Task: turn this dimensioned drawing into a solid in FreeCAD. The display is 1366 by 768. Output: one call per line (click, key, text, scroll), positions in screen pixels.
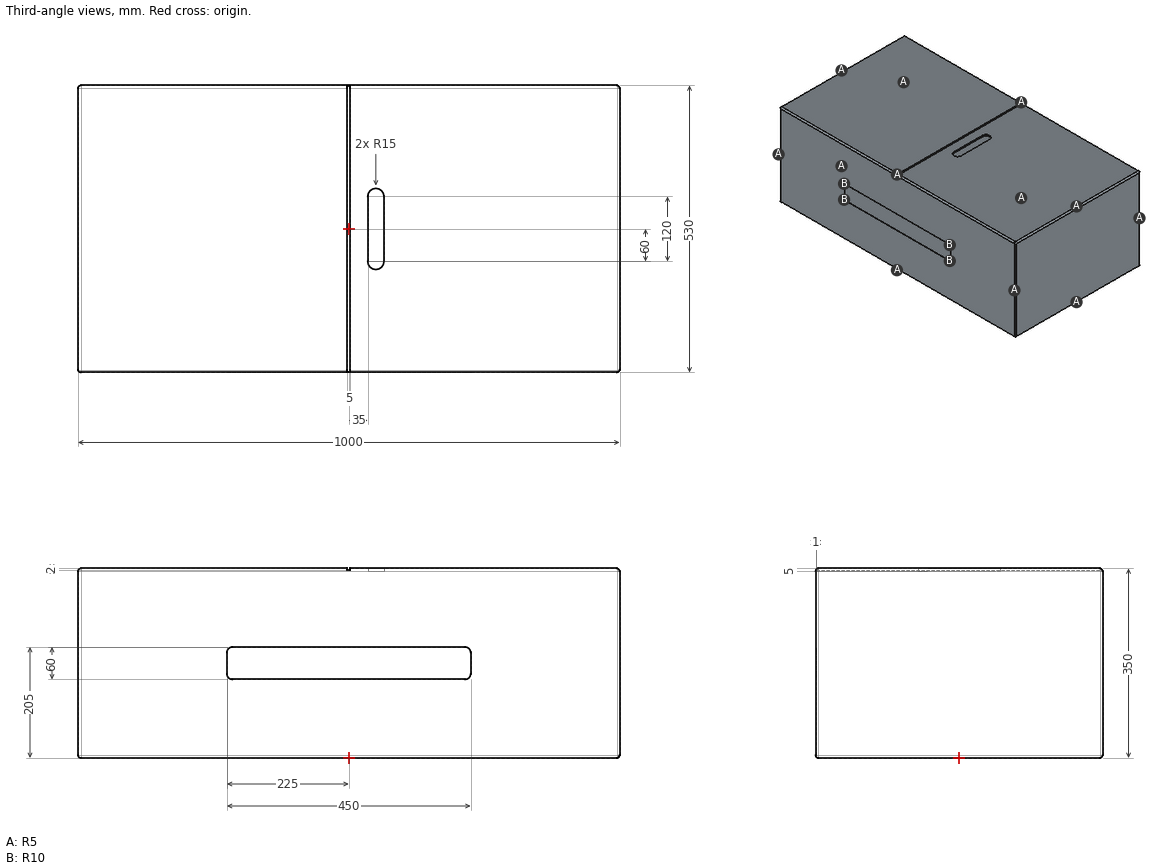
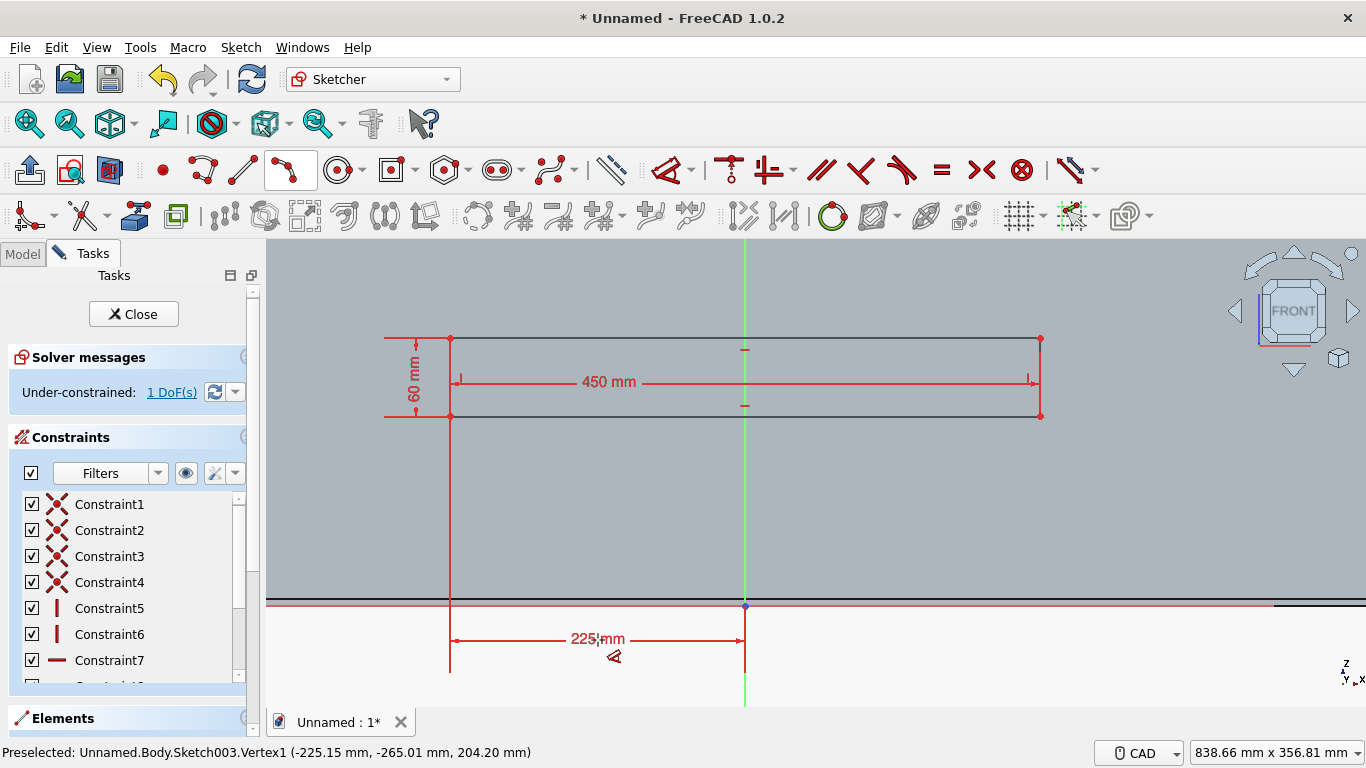
click(450, 338)
click(416, 472)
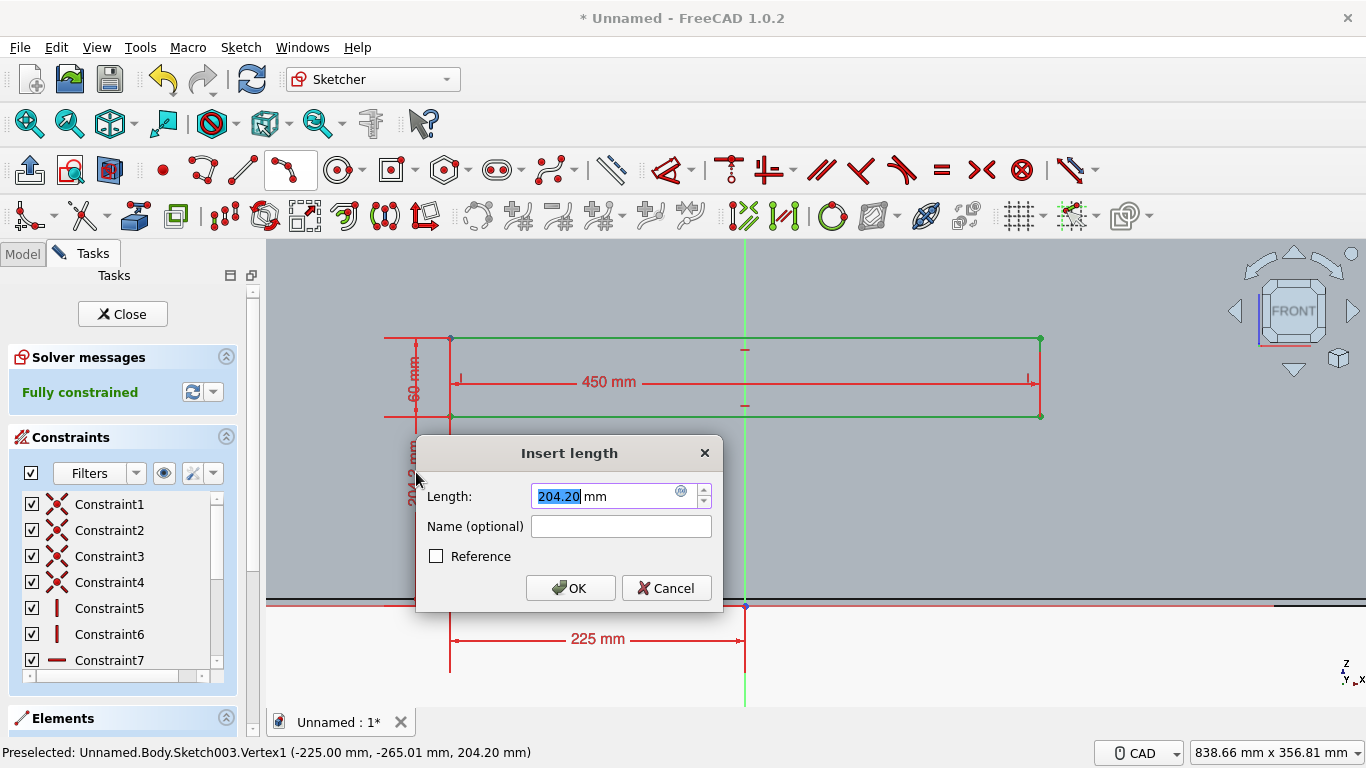
text(205)
key(Return)
key(Escape)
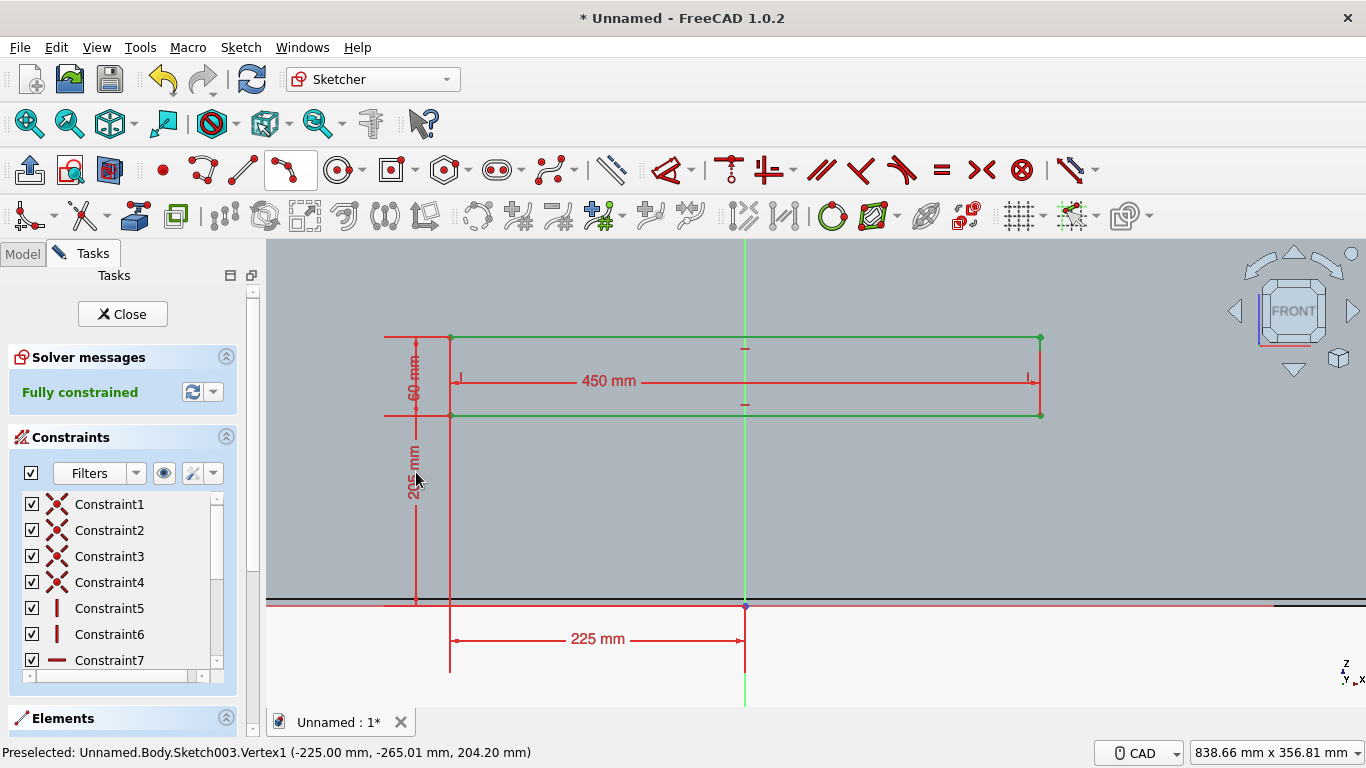
click(123, 314)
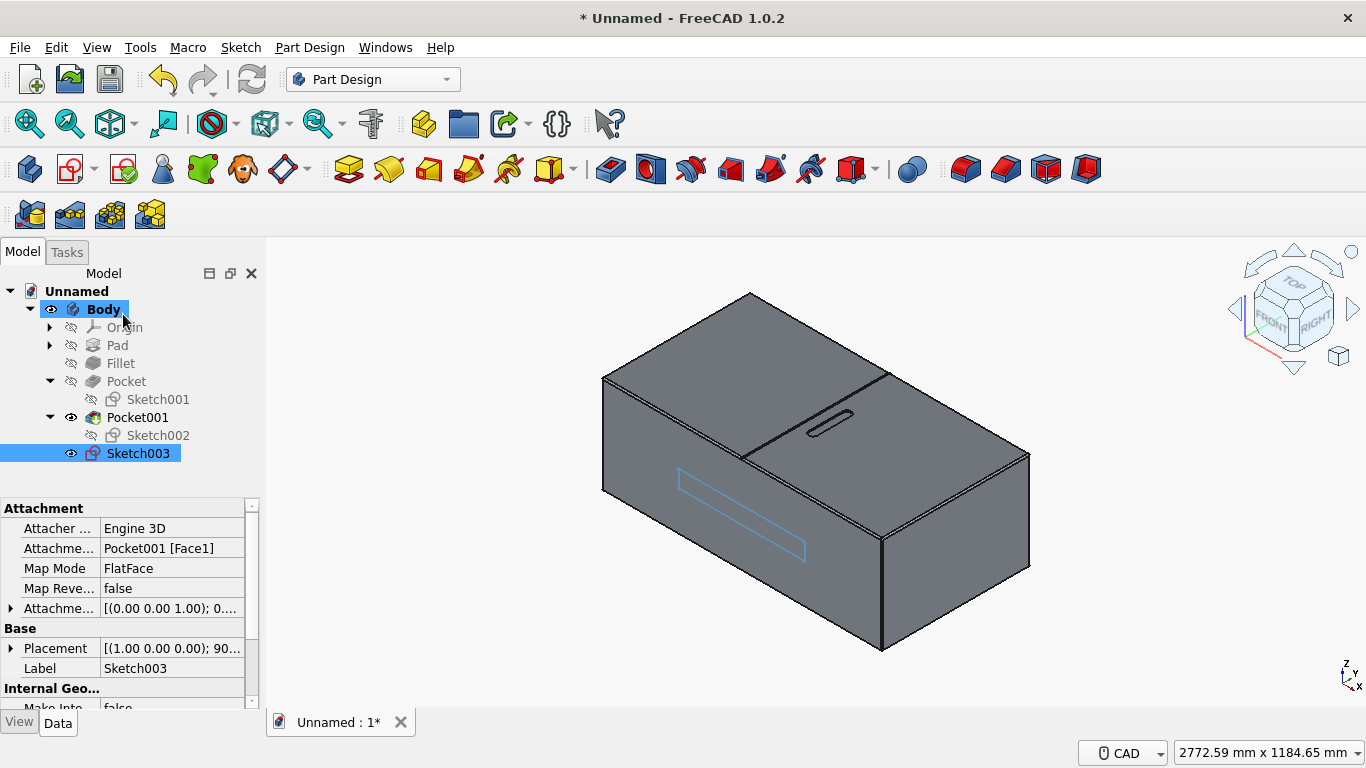
click(612, 170)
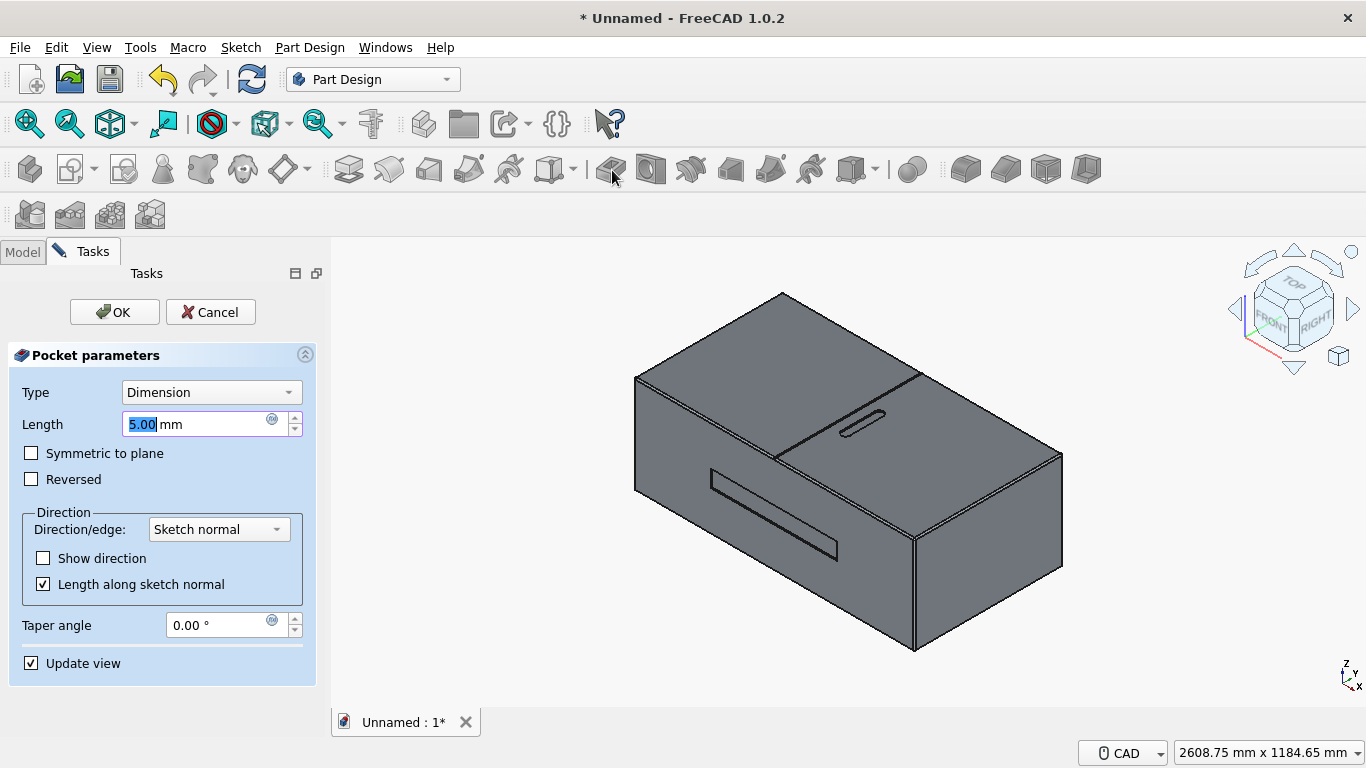
text(1)
key(Tab)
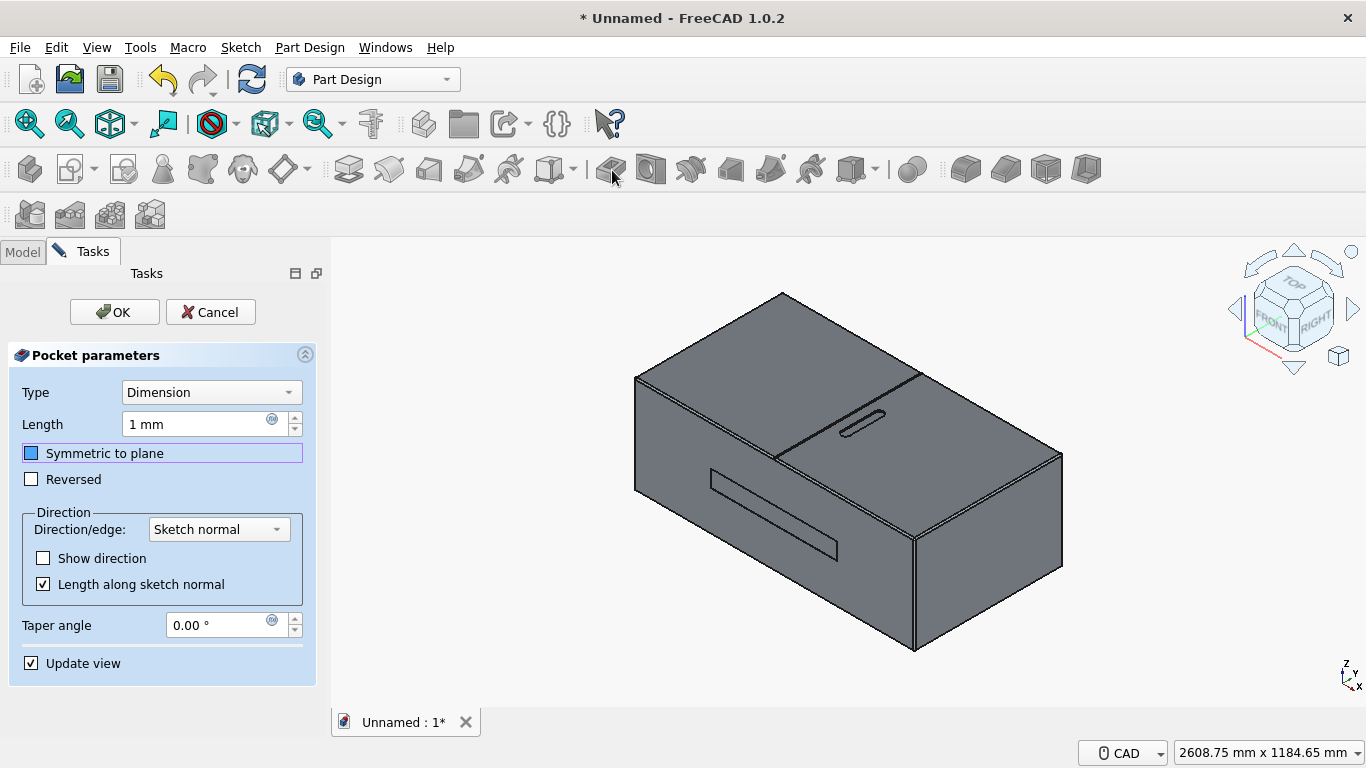
click(115, 312)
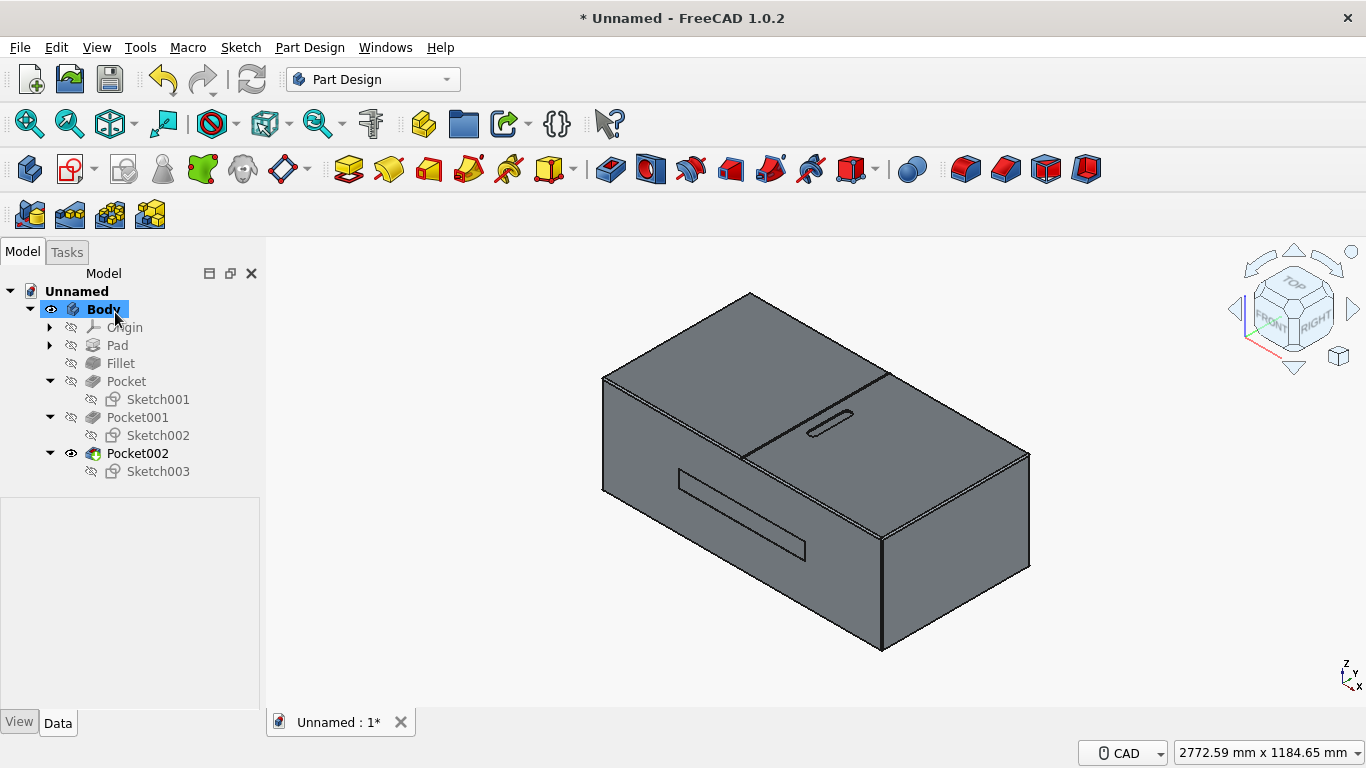
scroll(805, 541, up, 15)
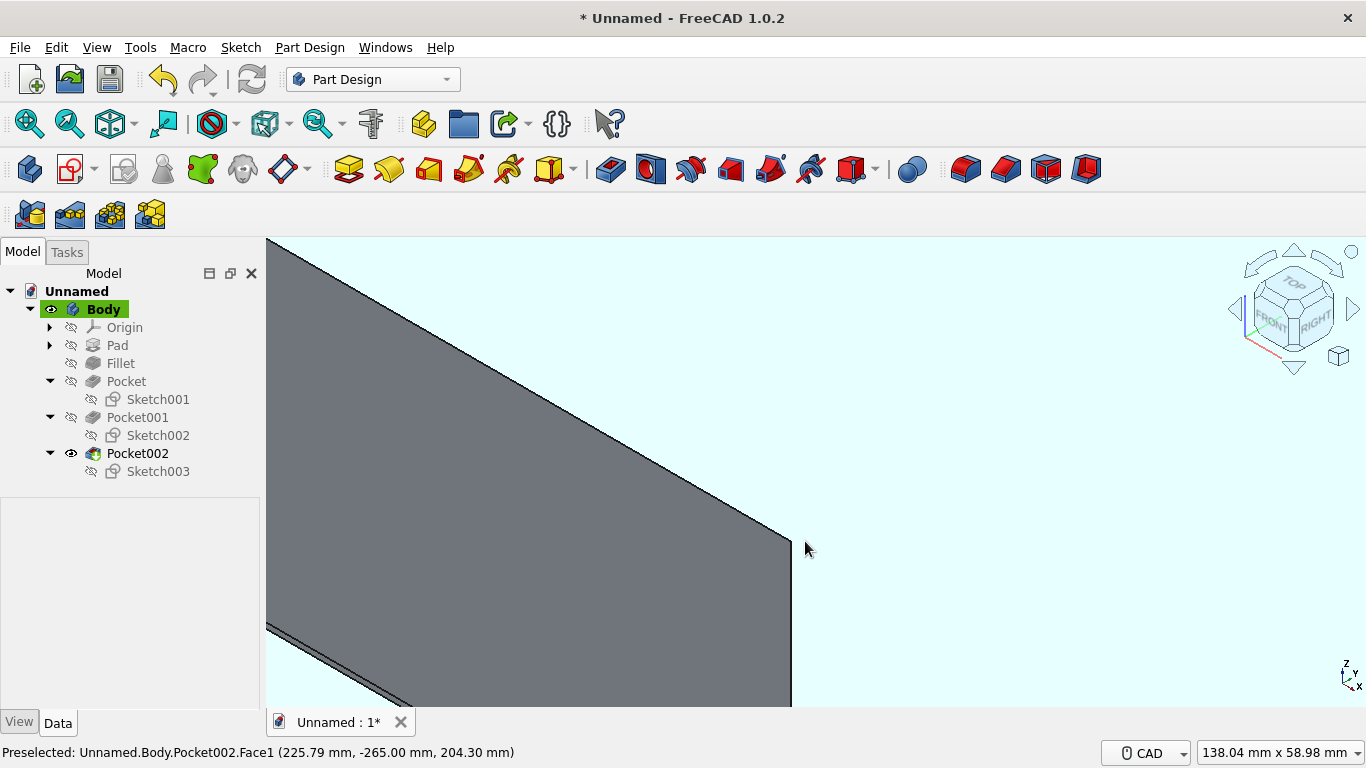
scroll(794, 539, up, 9)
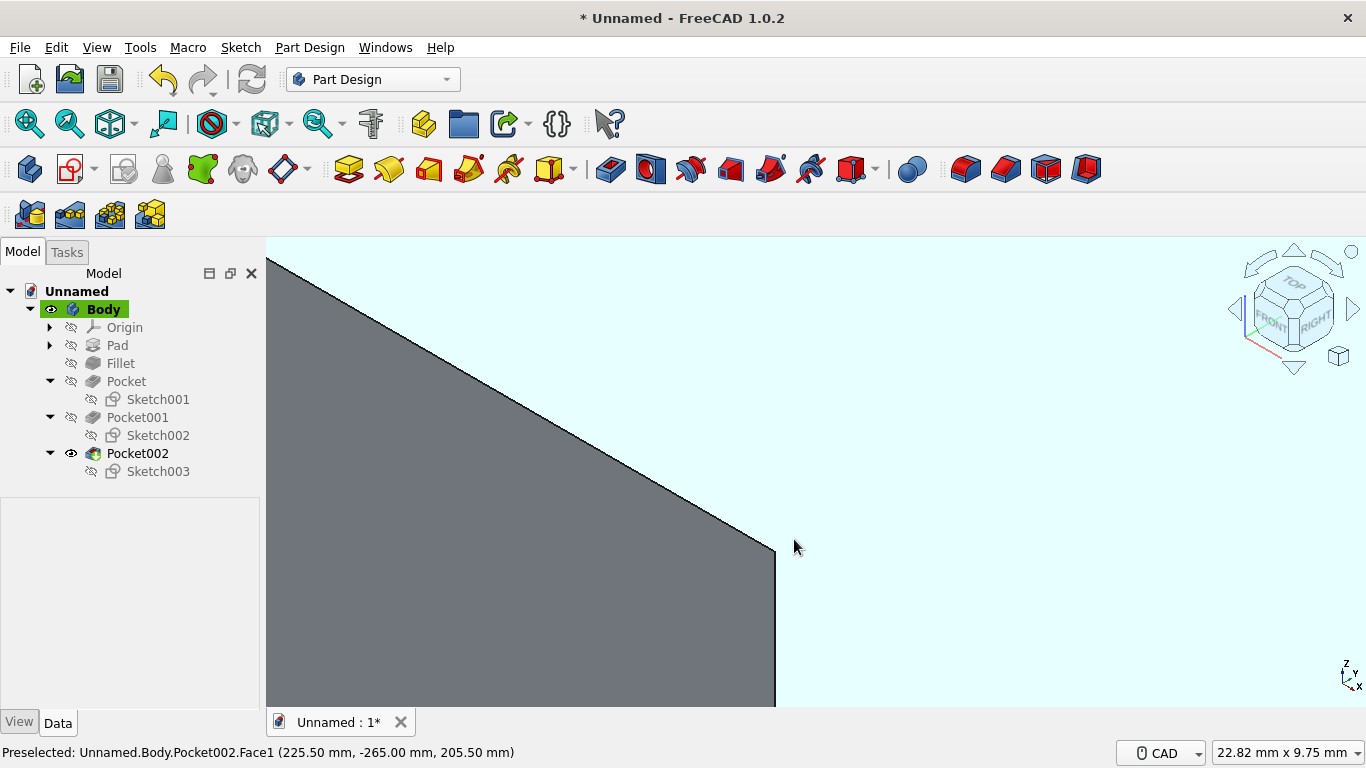
click(30, 124)